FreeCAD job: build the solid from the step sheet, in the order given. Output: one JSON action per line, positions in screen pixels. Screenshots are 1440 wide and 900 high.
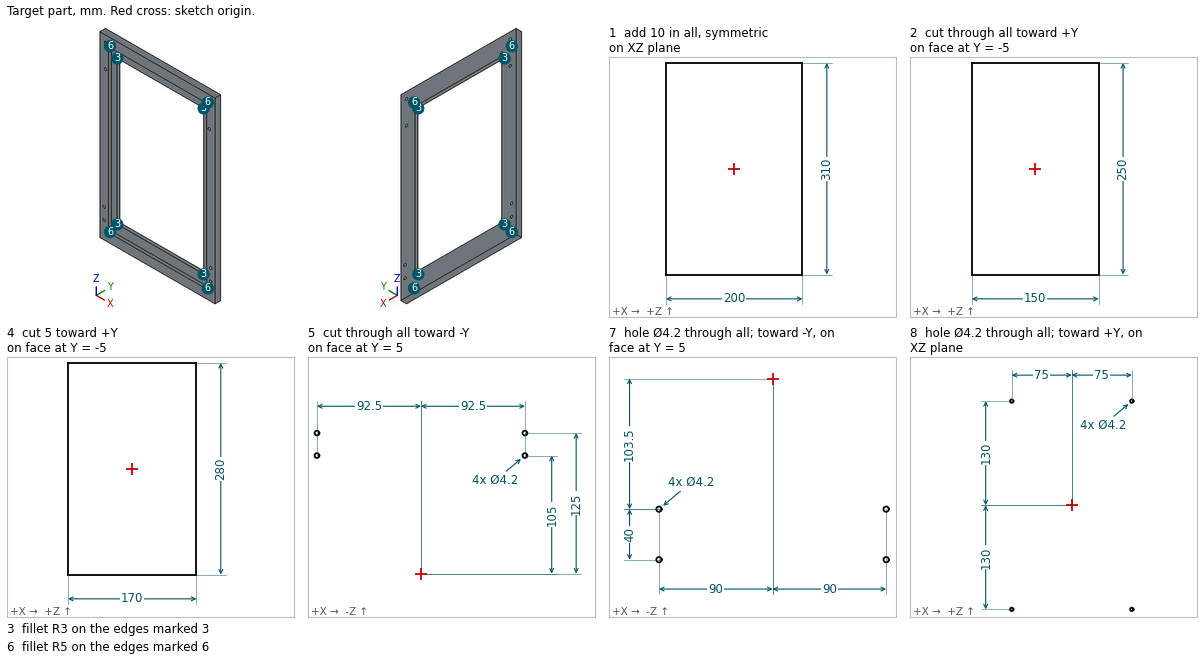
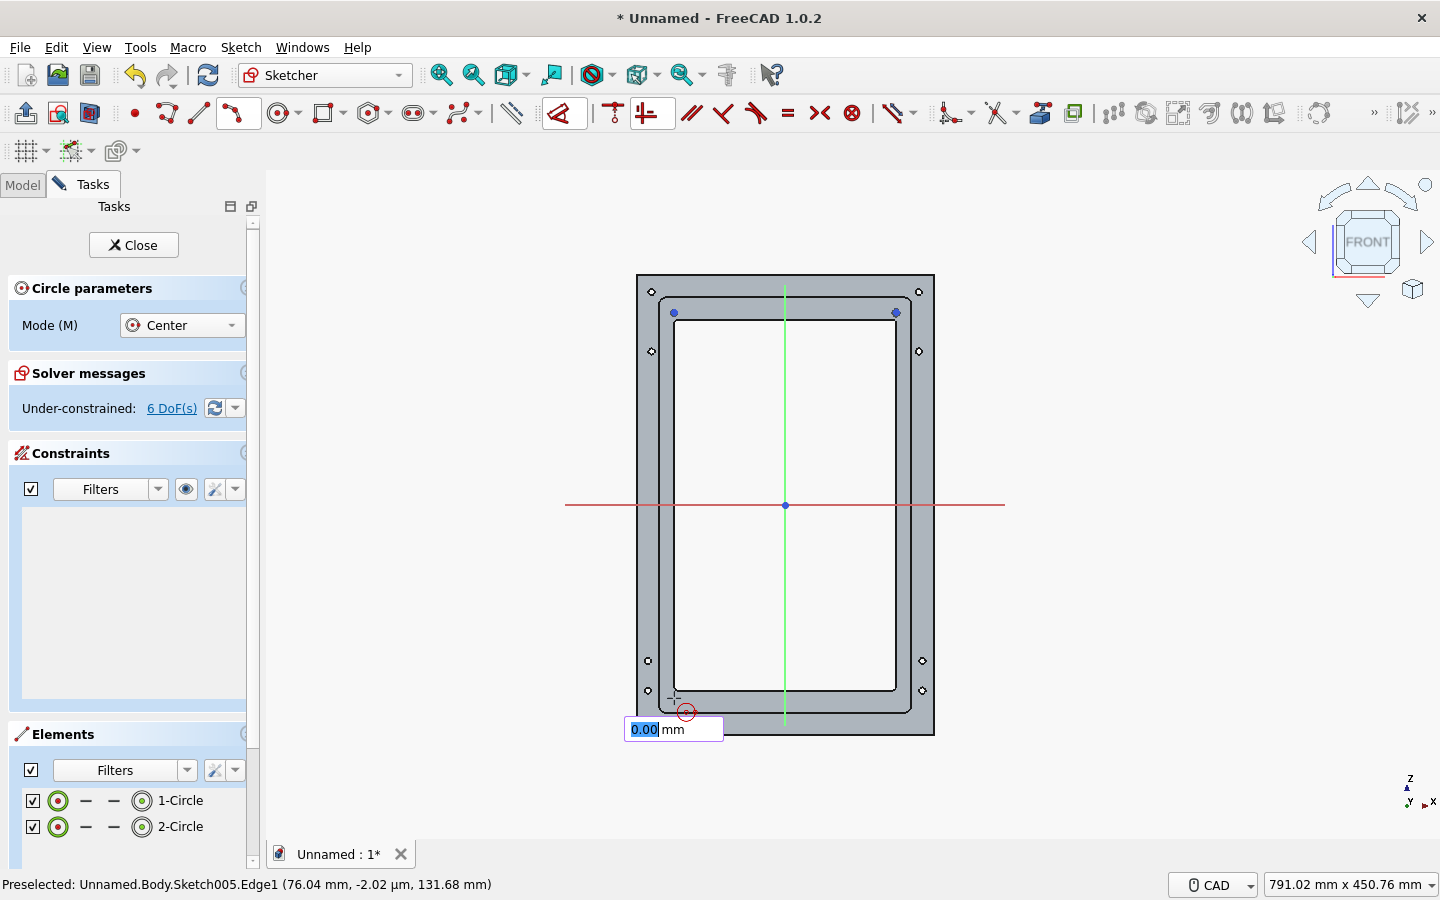
{"action": "scroll", "coordinate": [676, 696], "scroll_direction": "up", "scroll_amount": 9}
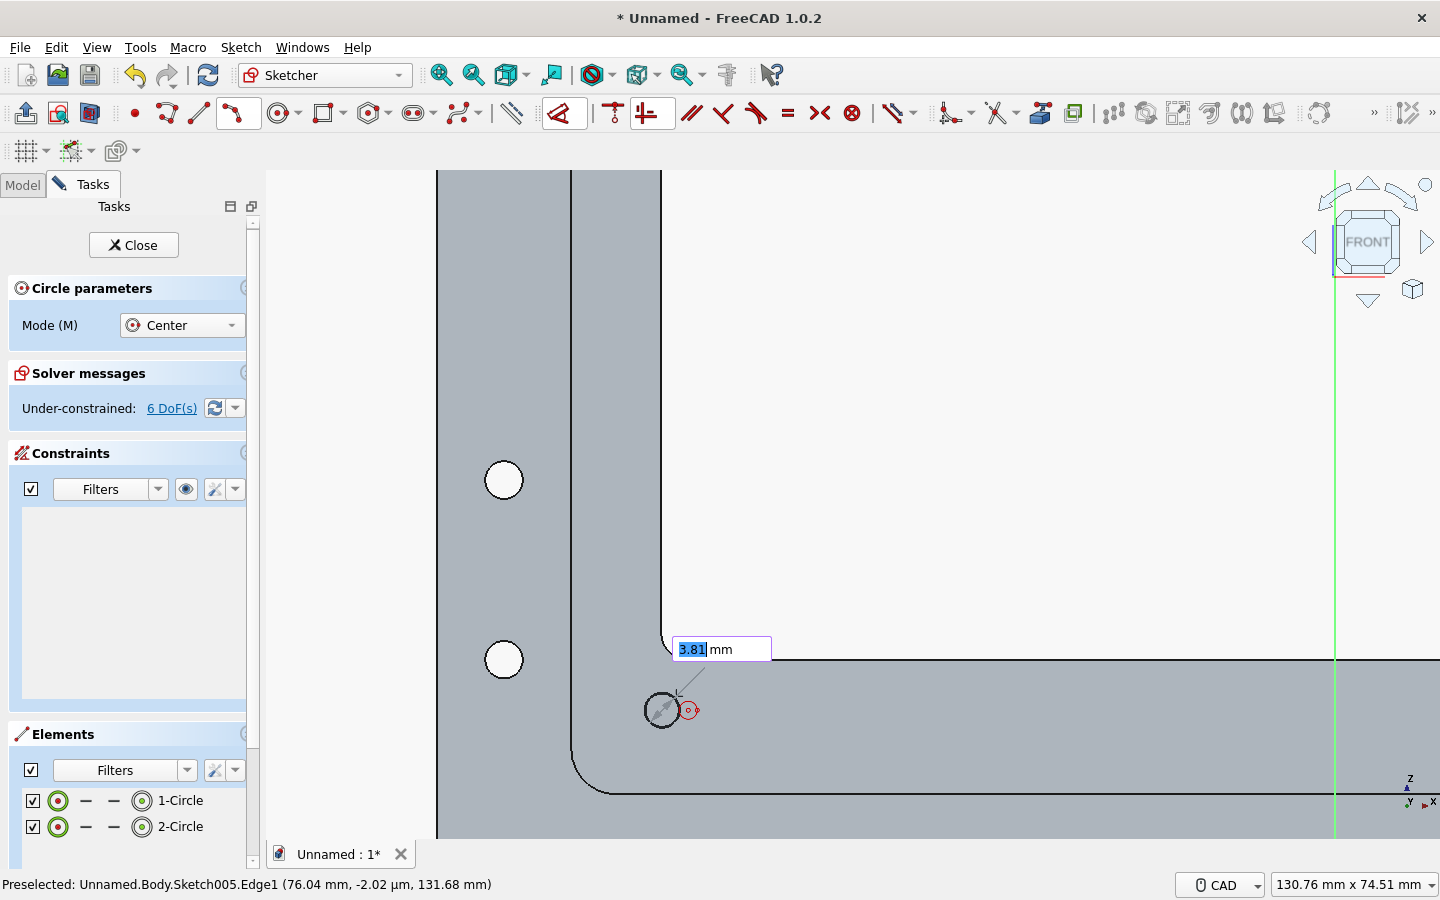
{"action": "left_click", "coordinate": [674, 691]}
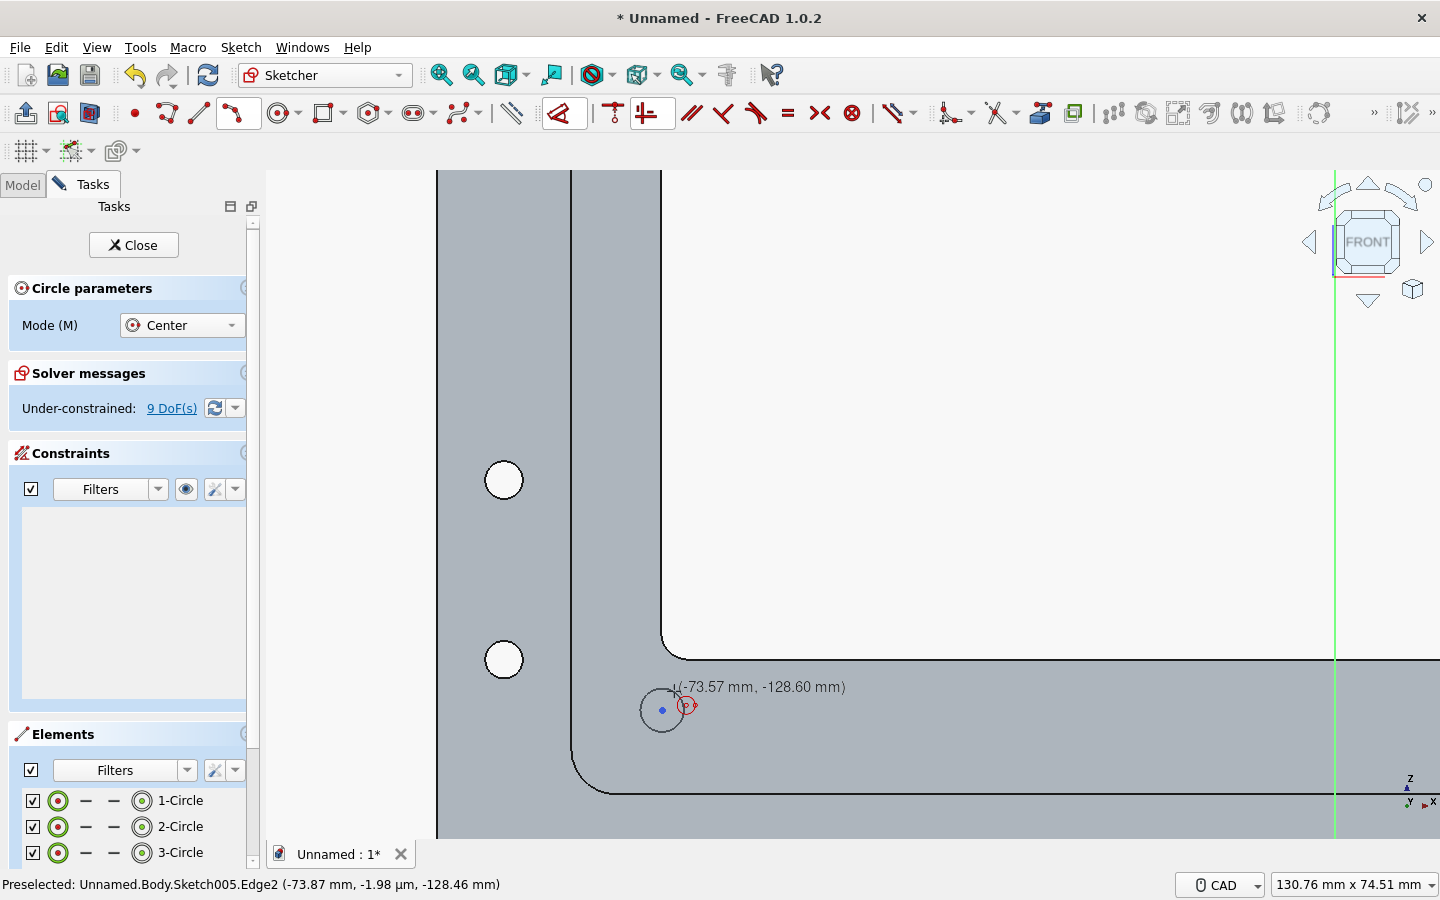
{"action": "scroll", "coordinate": [676, 696], "scroll_direction": "down", "scroll_amount": 9}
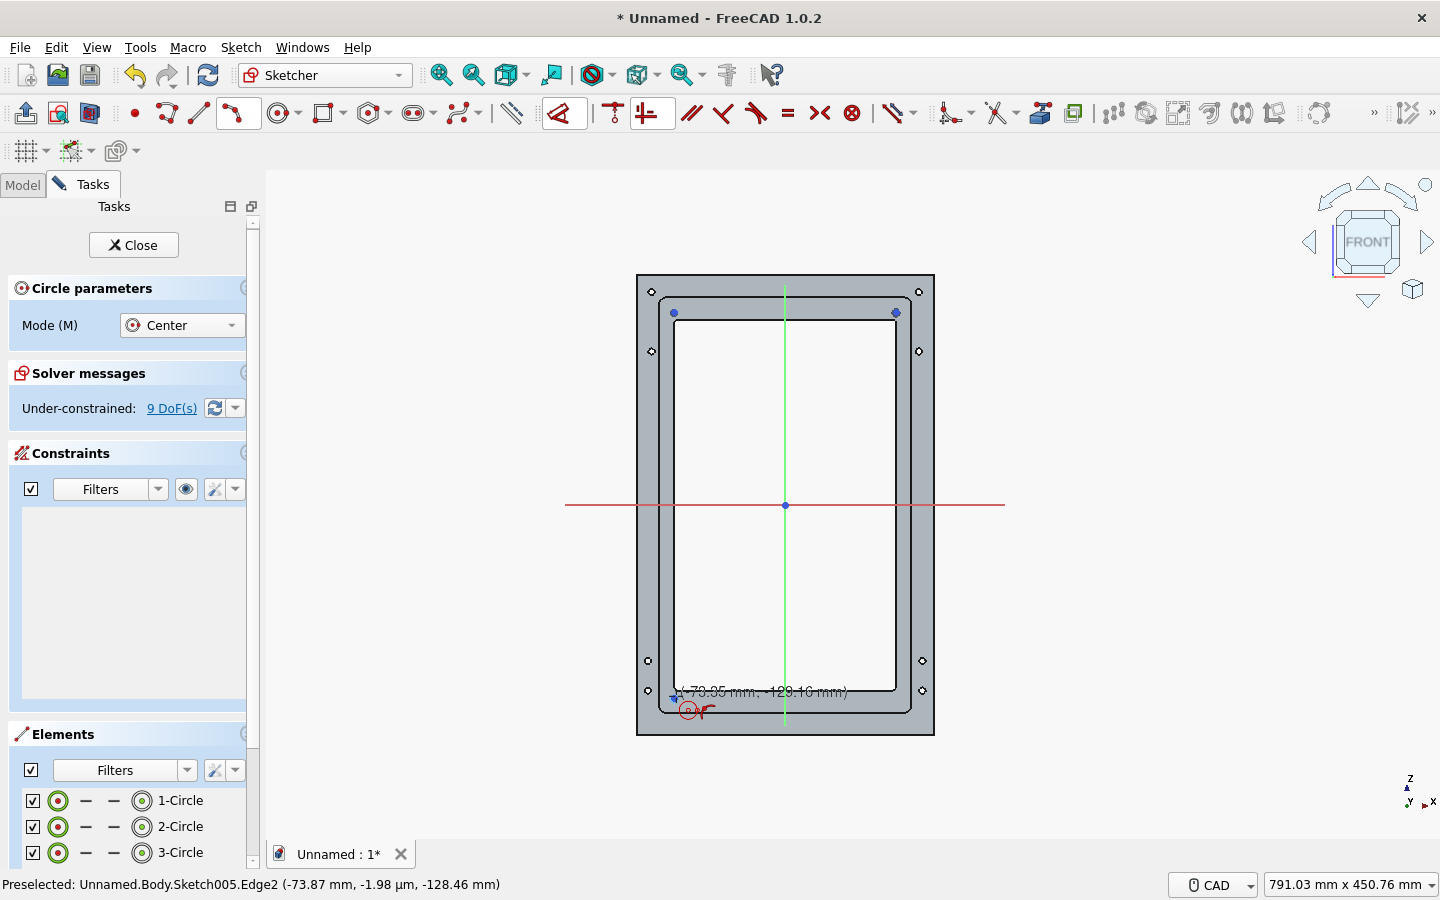
{"action": "scroll", "coordinate": [896, 698], "scroll_direction": "up", "scroll_amount": 10}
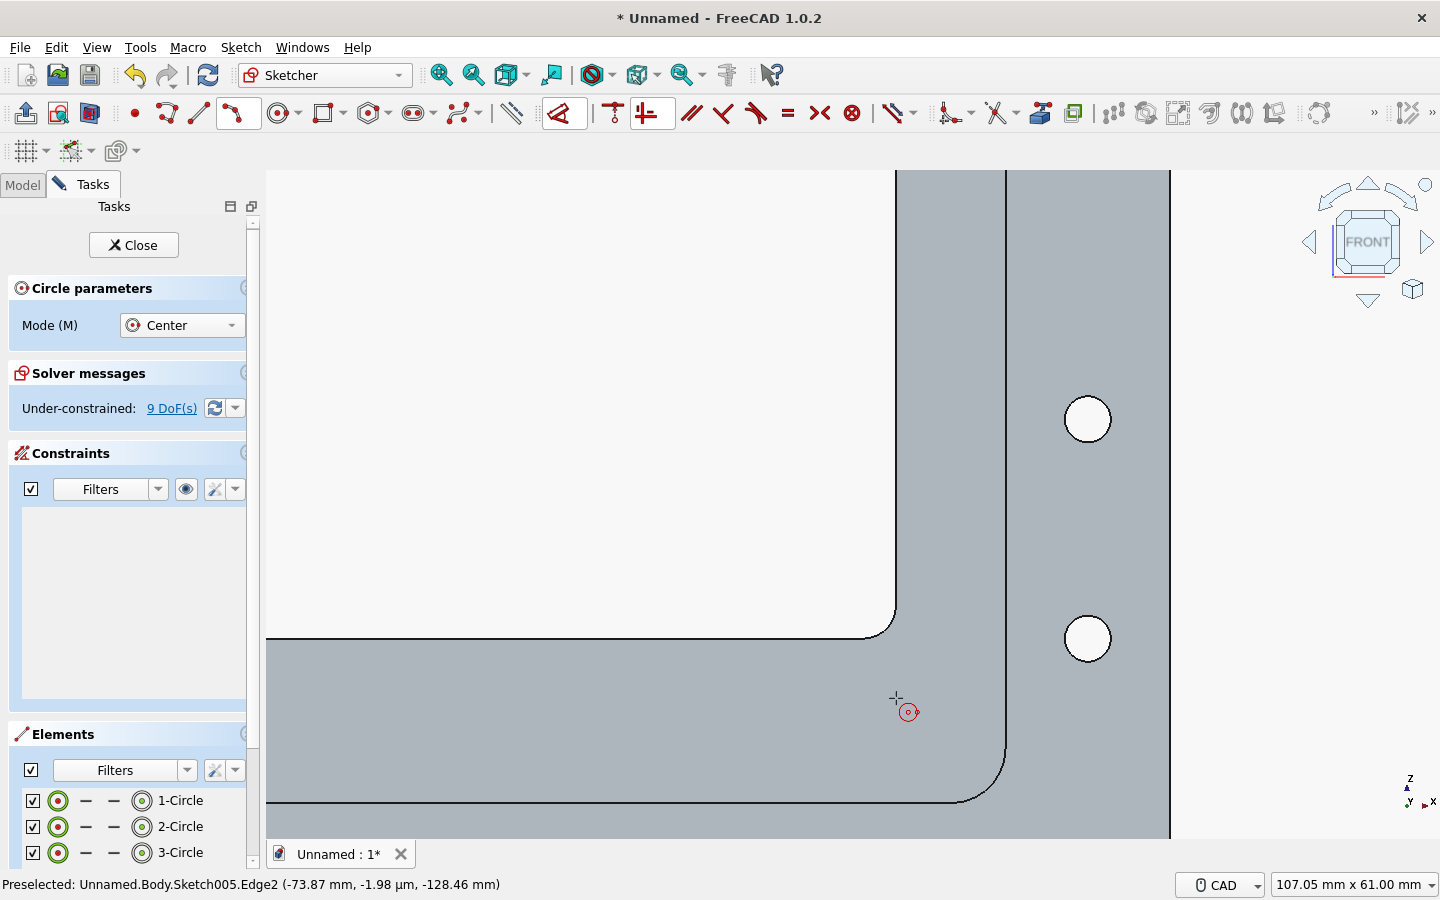
{"action": "scroll", "coordinate": [896, 698], "scroll_direction": "down", "scroll_amount": 10}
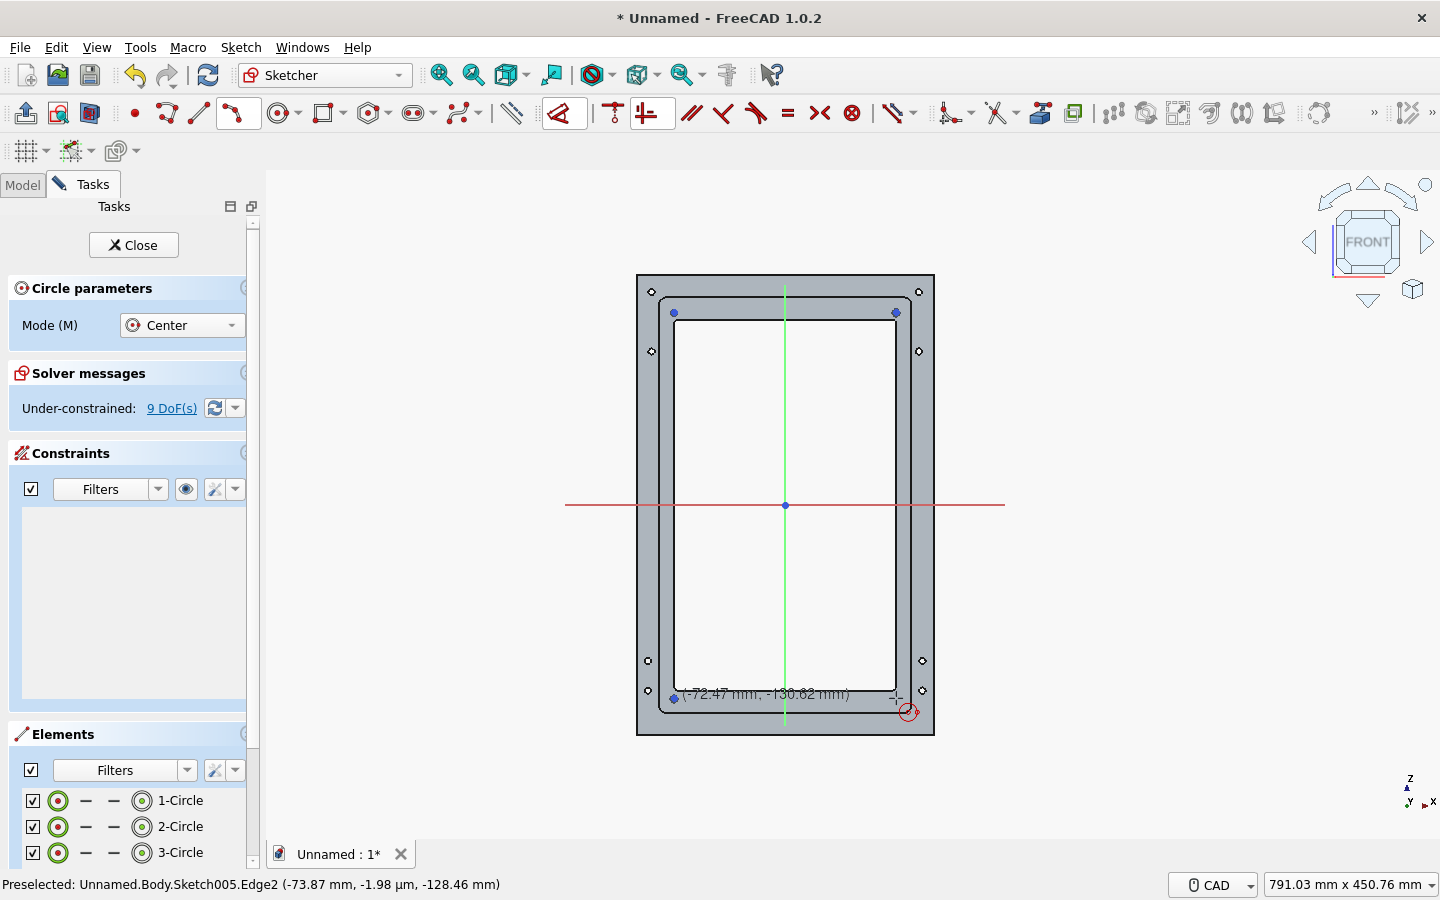
{"action": "left_click", "coordinate": [896, 698]}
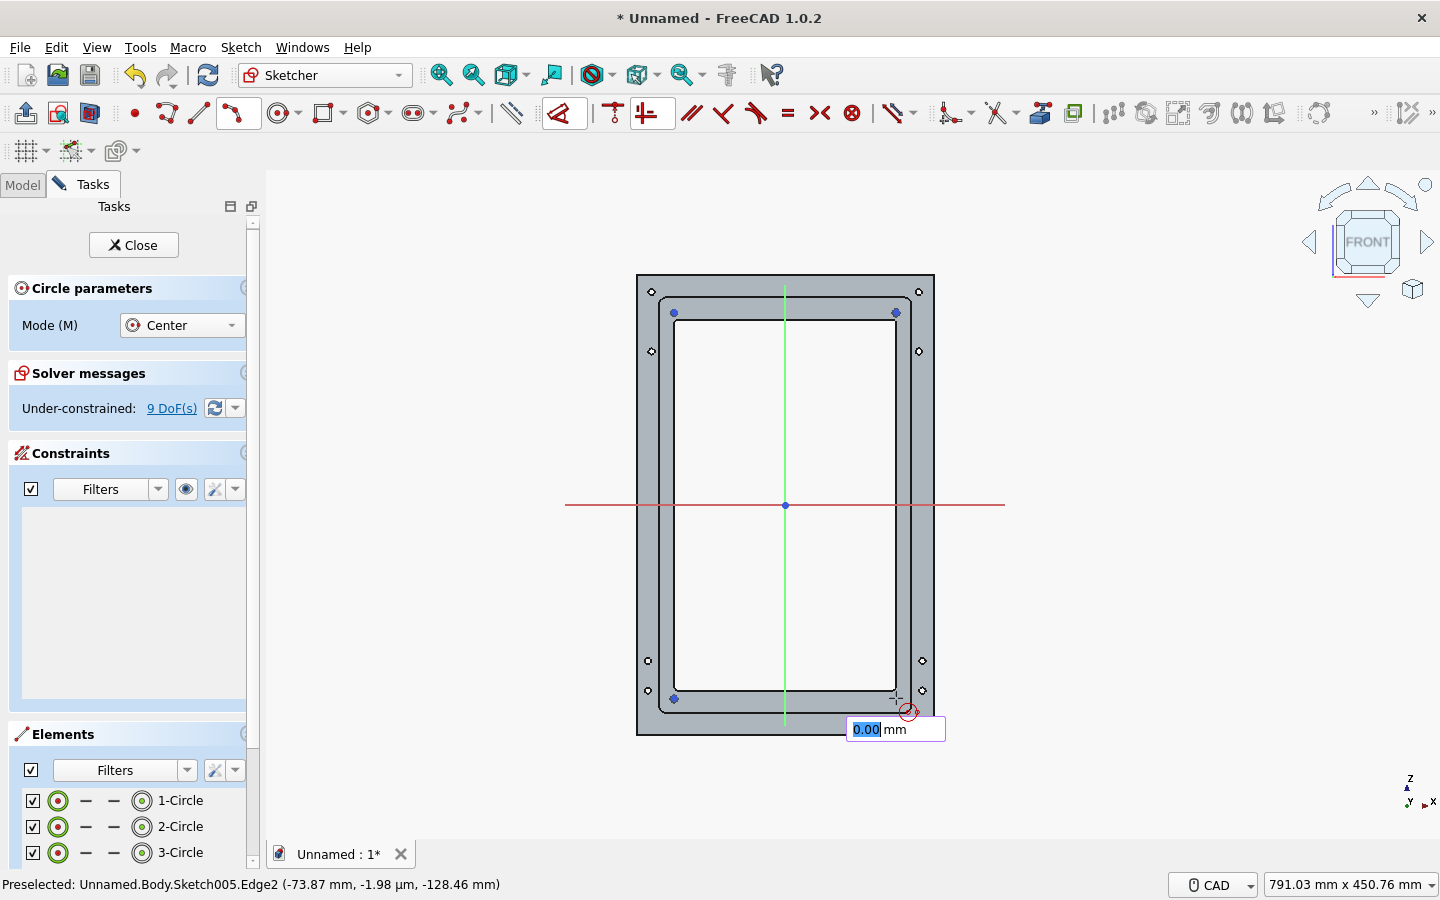
{"action": "scroll", "coordinate": [899, 696], "scroll_direction": "up", "scroll_amount": 9}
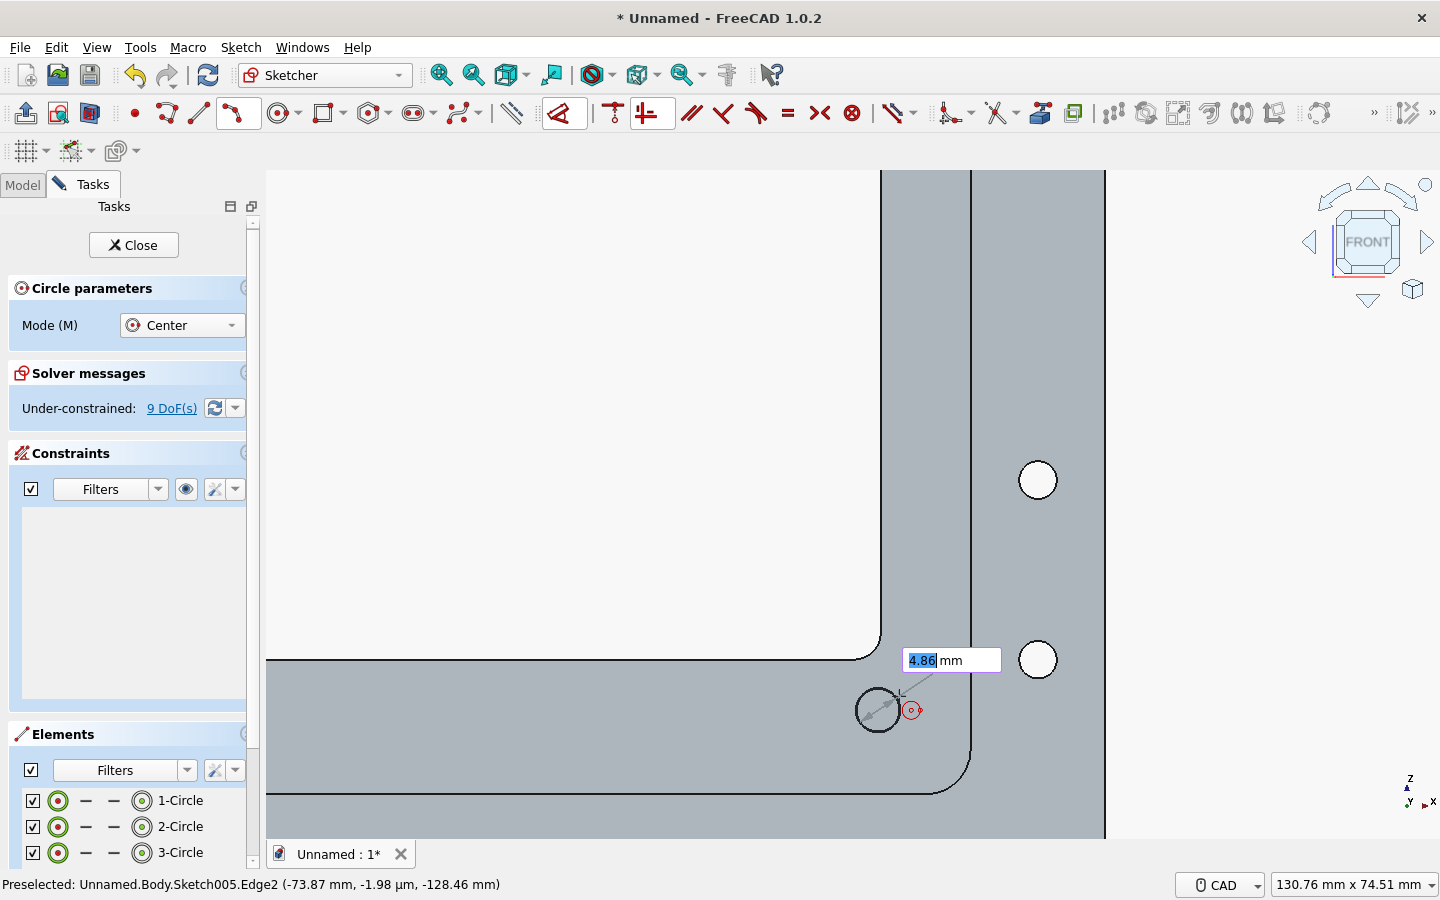
{"action": "left_click", "coordinate": [894, 691]}
{"action": "key", "text": "Escape"}